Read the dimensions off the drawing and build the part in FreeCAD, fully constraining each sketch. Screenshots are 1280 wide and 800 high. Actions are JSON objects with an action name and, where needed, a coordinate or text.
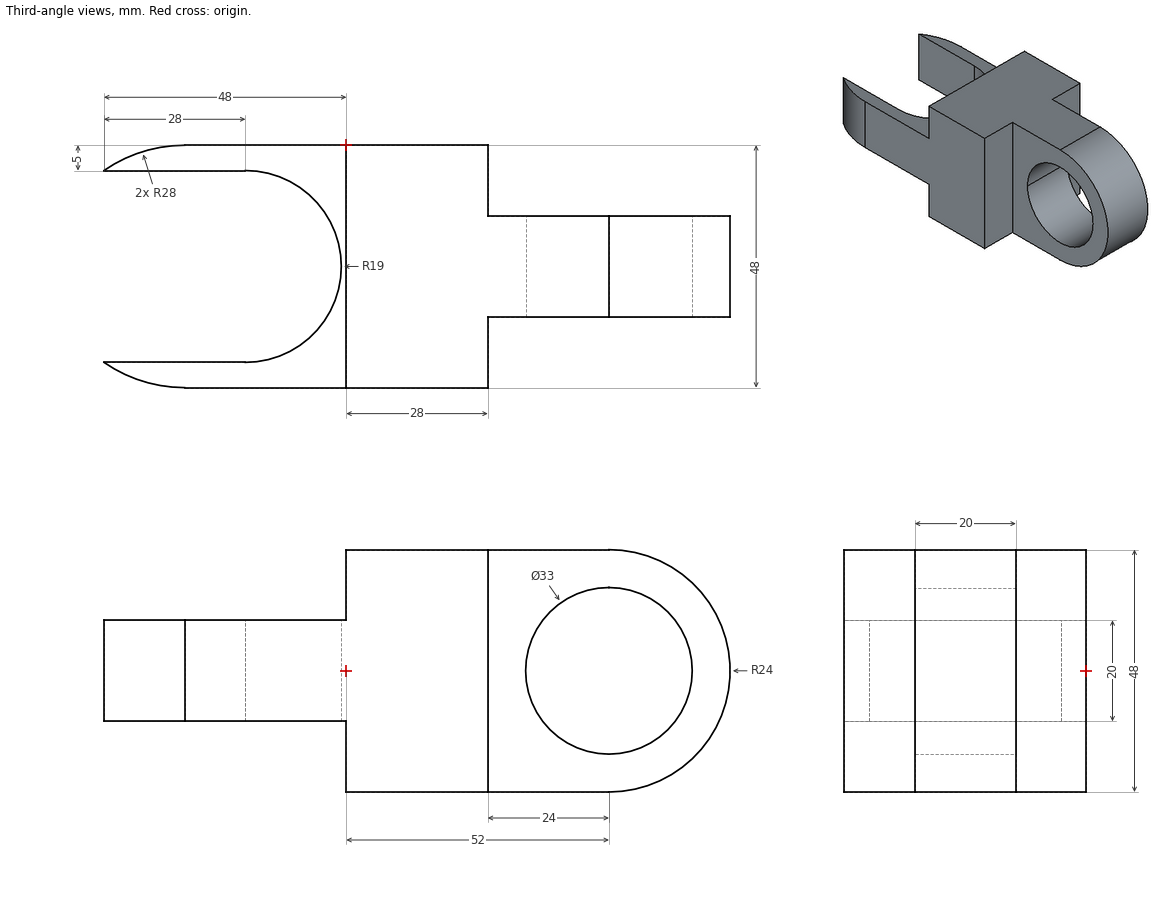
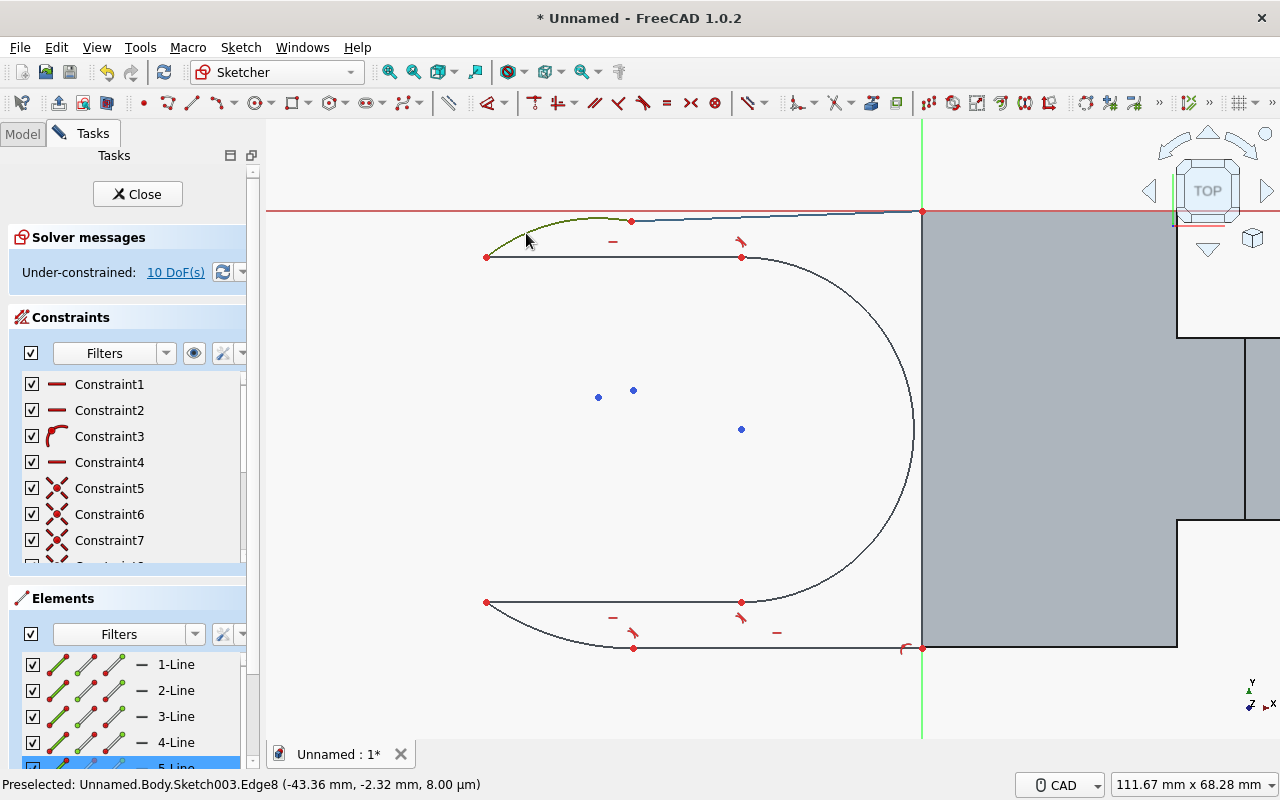
{"action": "left_click", "coordinate": [644, 104]}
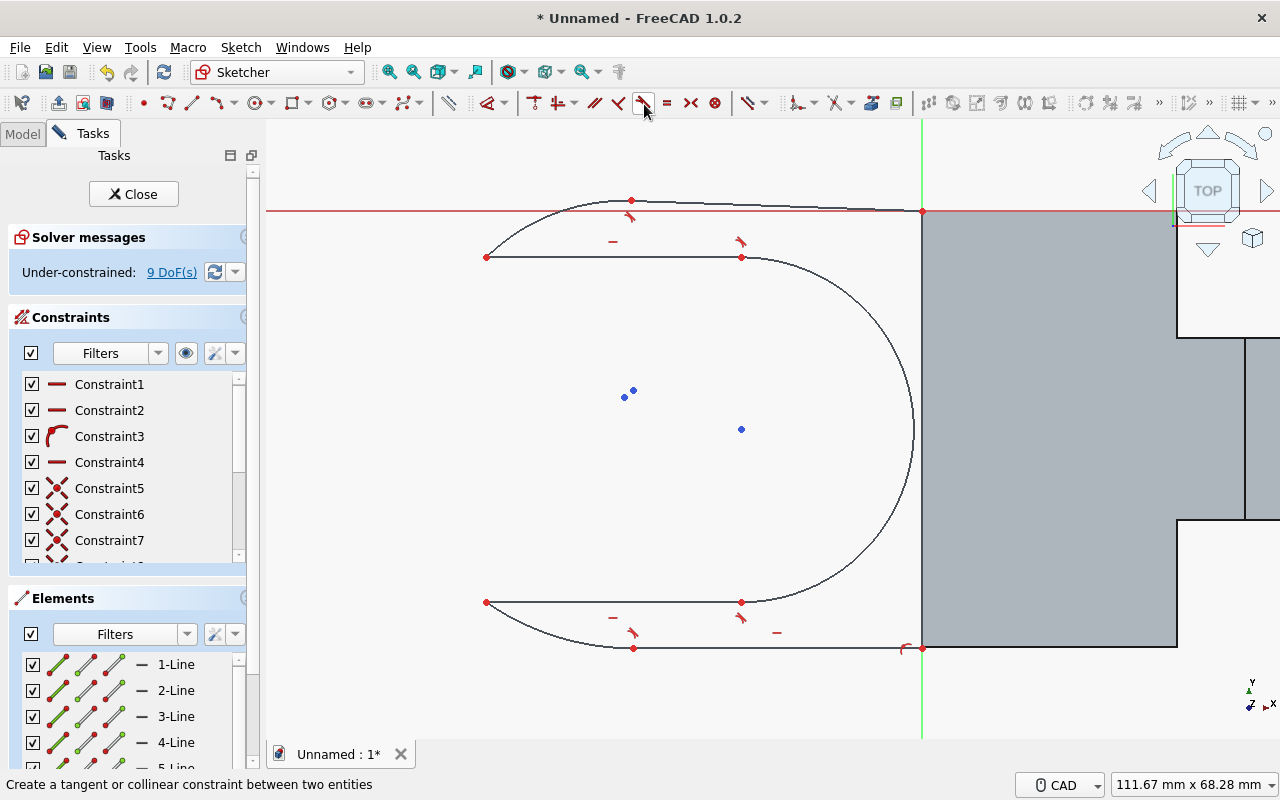
{"action": "left_click", "coordinate": [835, 208]}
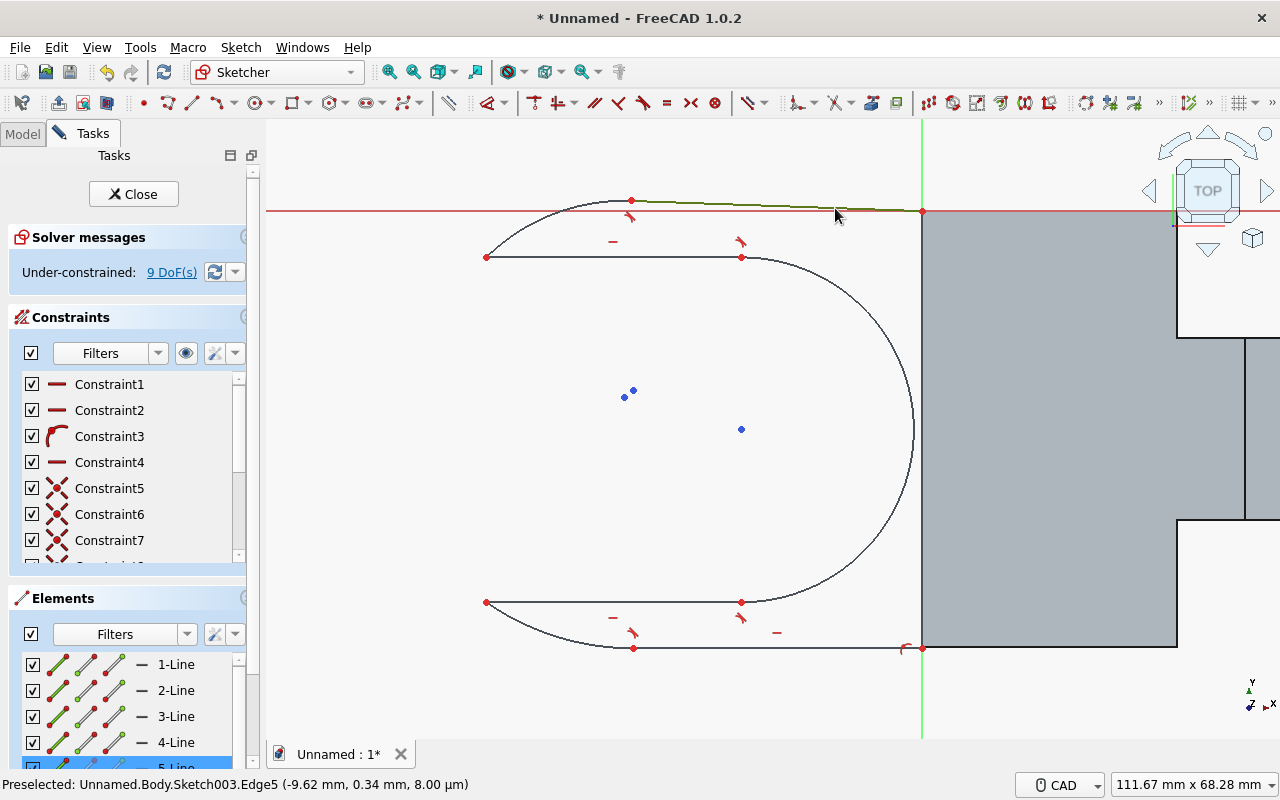
{"action": "key", "text": "h"}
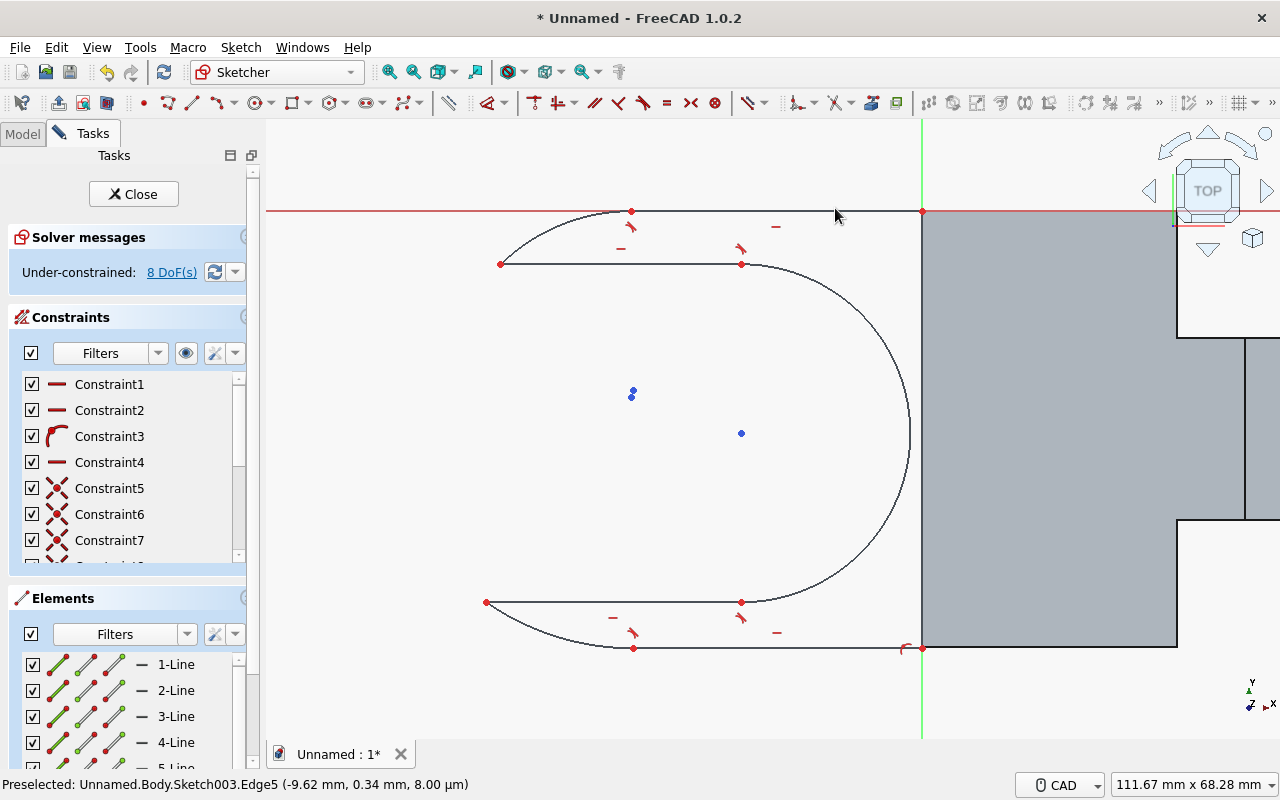
{"action": "left_click", "coordinate": [527, 625]}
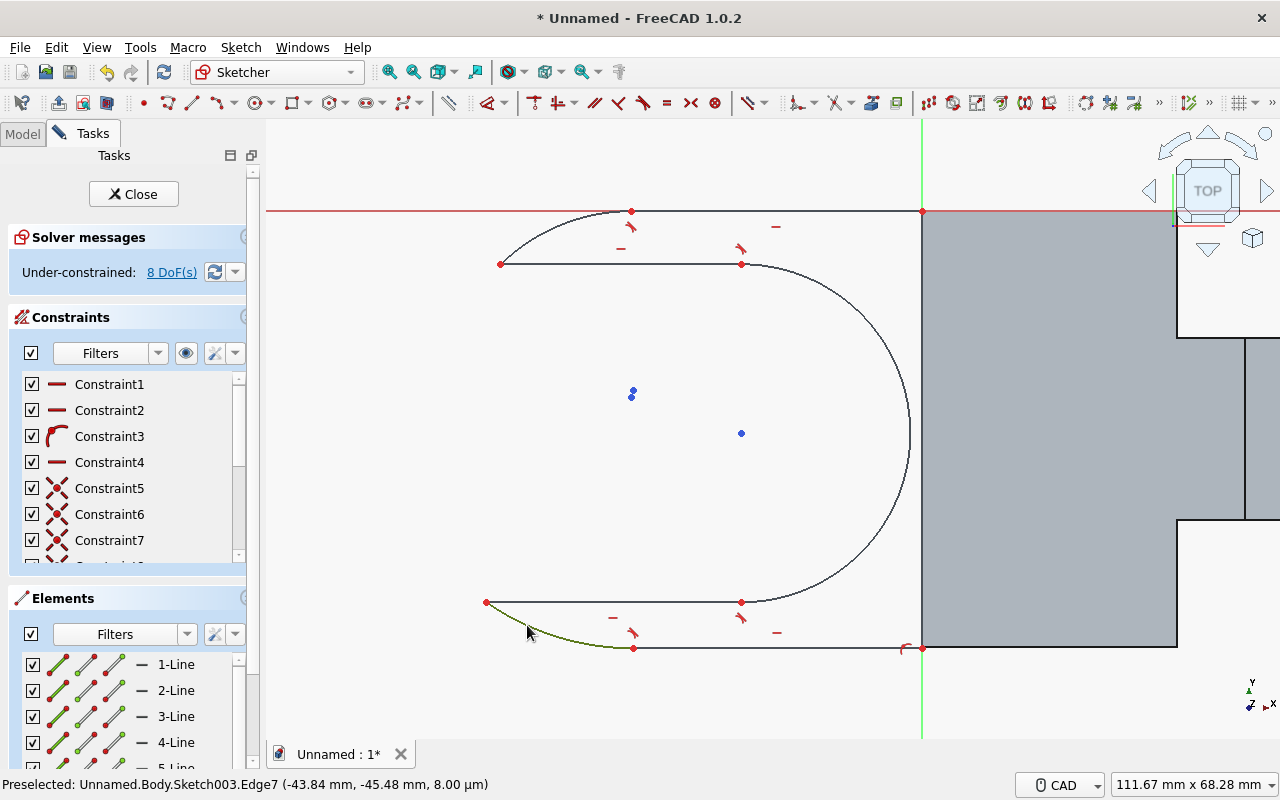
{"action": "left_click", "coordinate": [535, 238]}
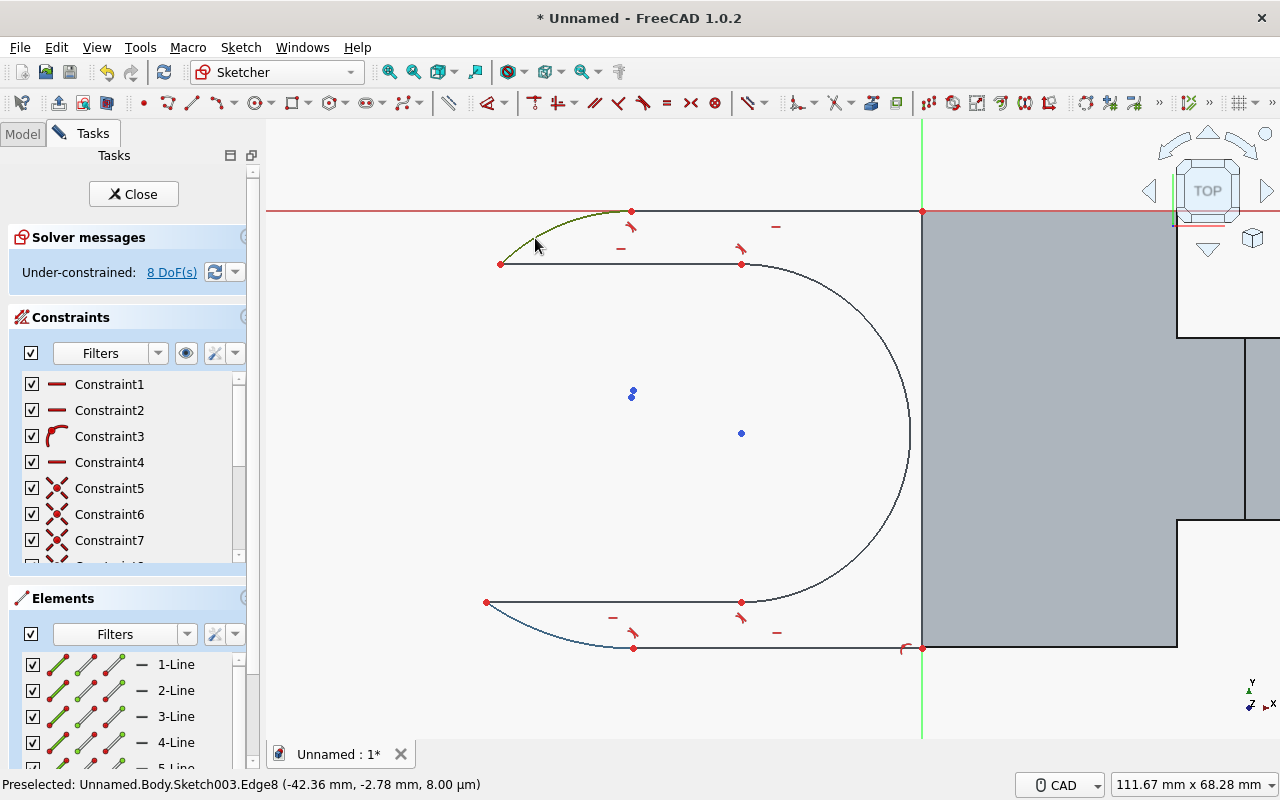
{"action": "key", "text": "e"}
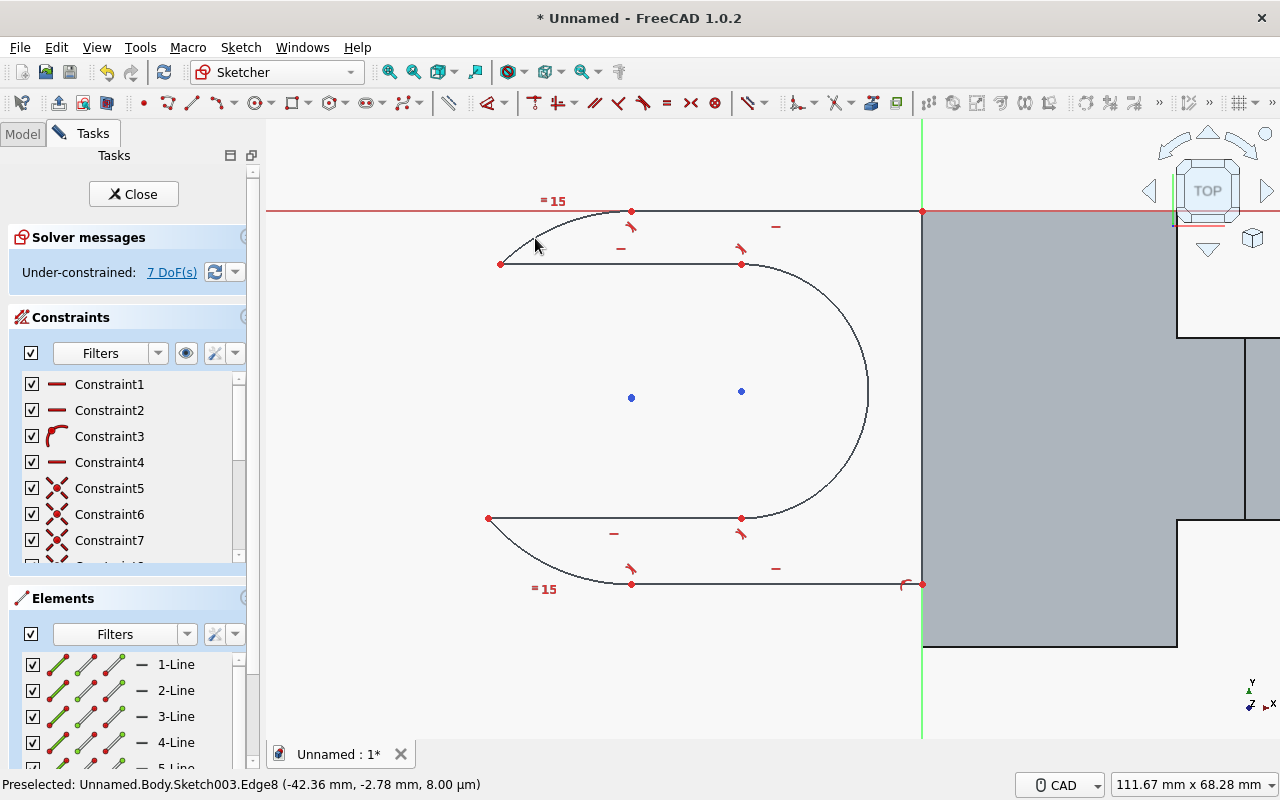
{"action": "left_click", "coordinate": [488, 104]}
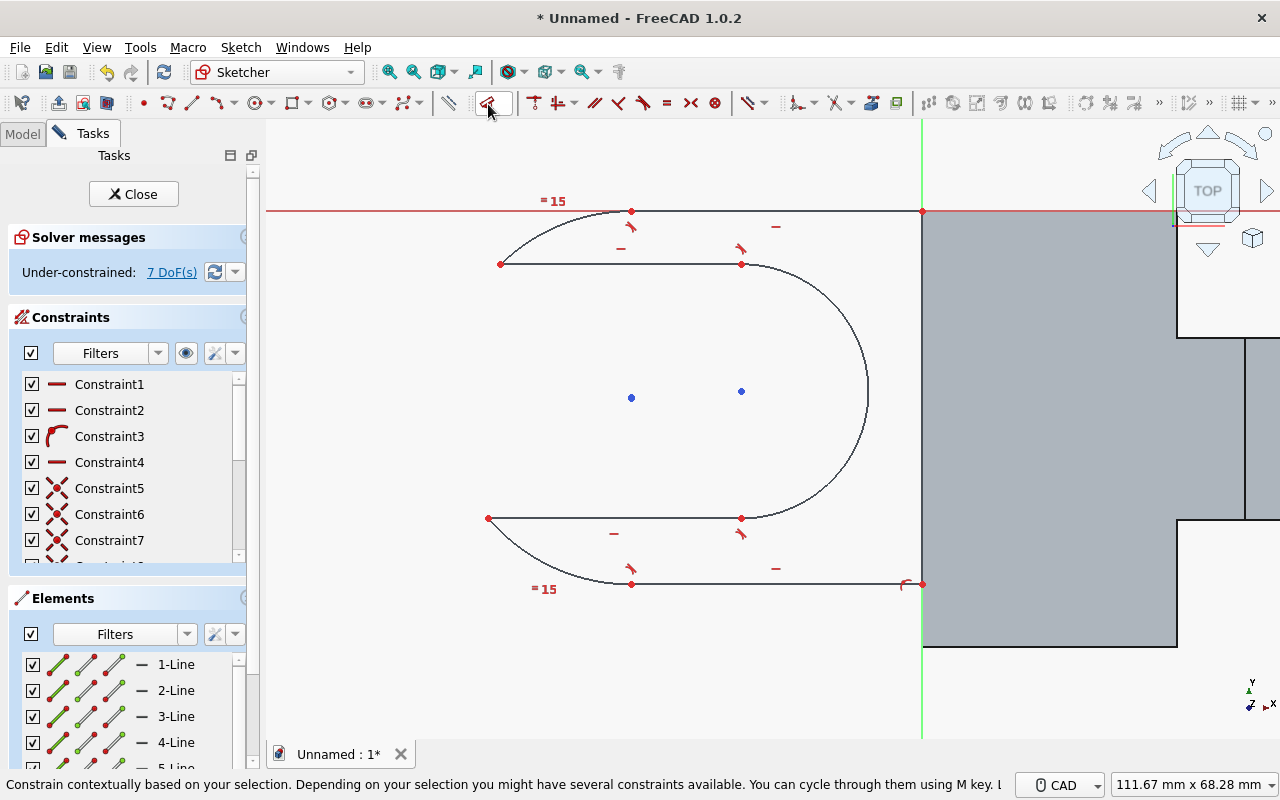
{"action": "left_click", "coordinate": [844, 466]}
{"action": "left_click", "coordinate": [870, 485]}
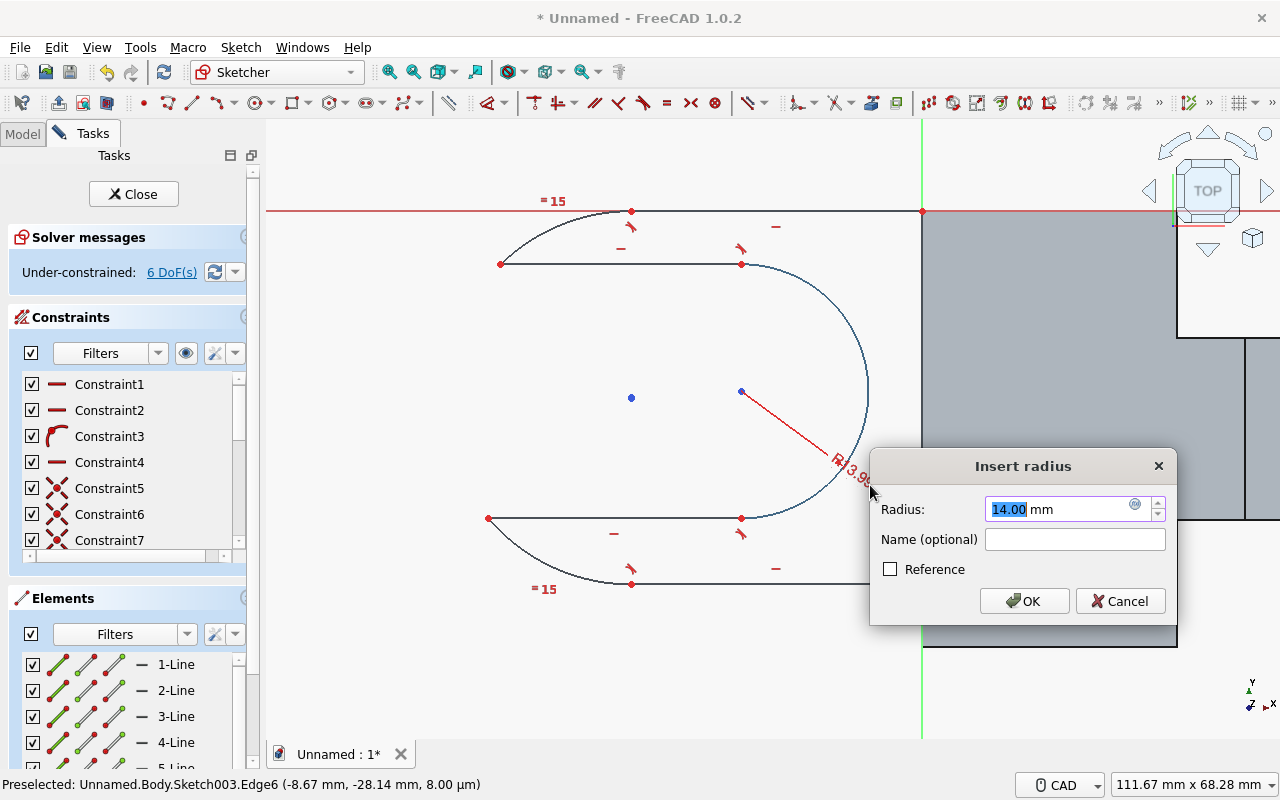
{"action": "type", "text": "19"}
{"action": "key", "text": "Return"}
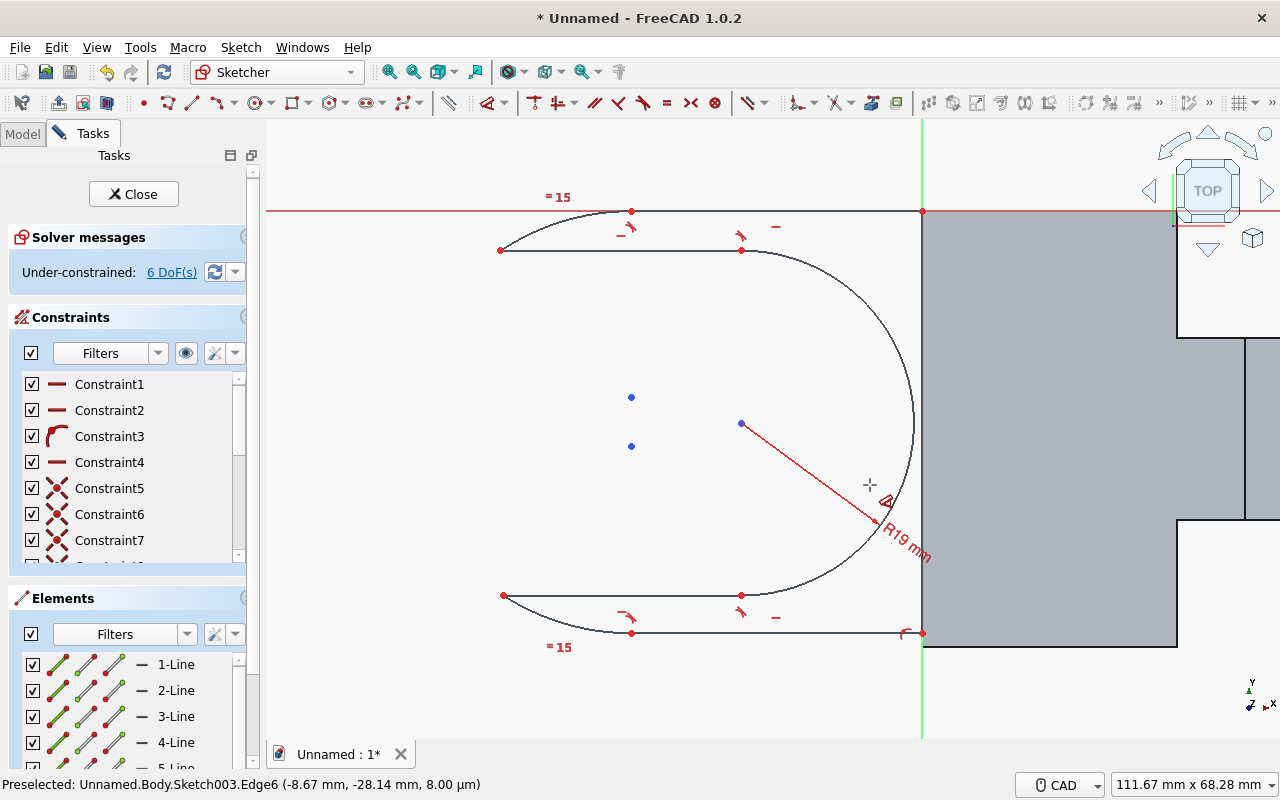
{"action": "left_click", "coordinate": [539, 615]}
{"action": "left_click", "coordinate": [527, 644]}